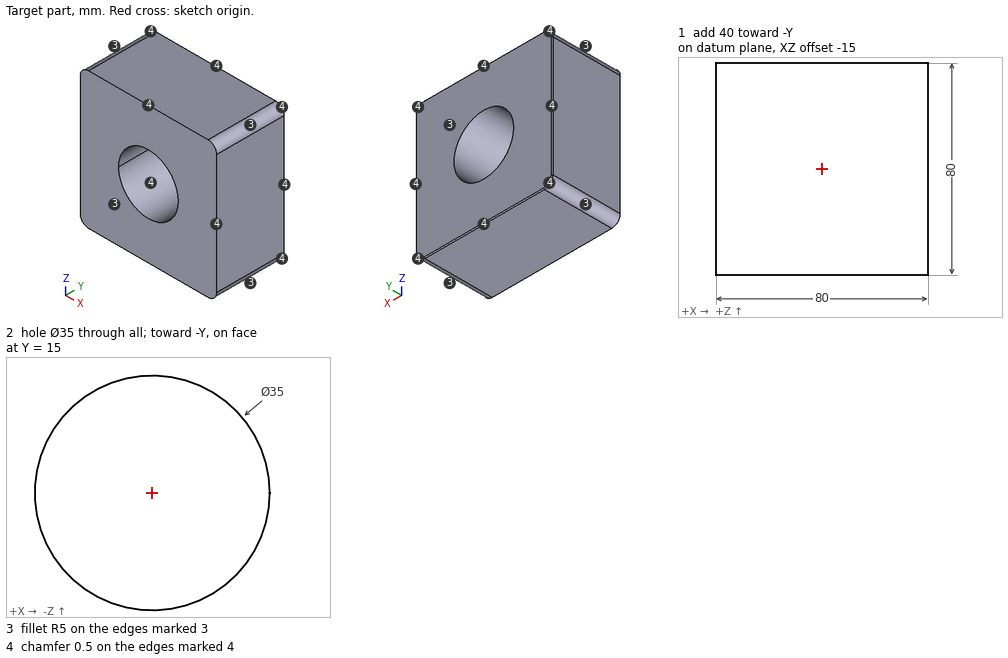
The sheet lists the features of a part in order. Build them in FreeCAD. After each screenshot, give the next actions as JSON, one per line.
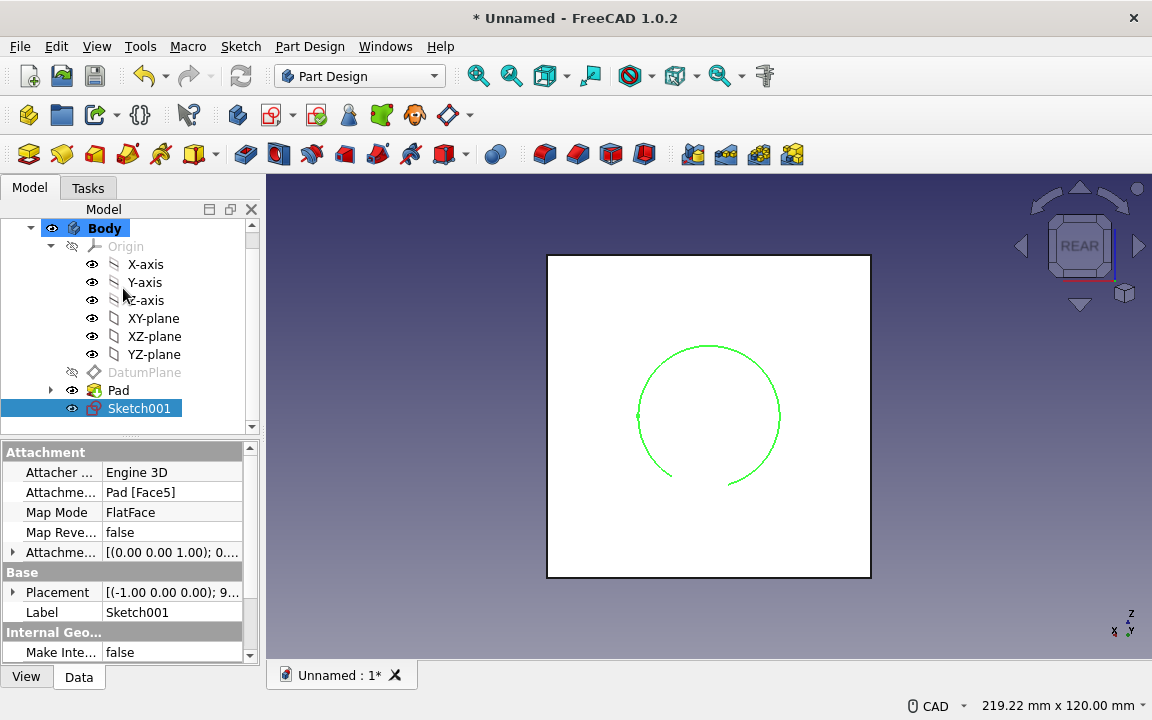
{"action": "left_click", "coordinate": [279, 154]}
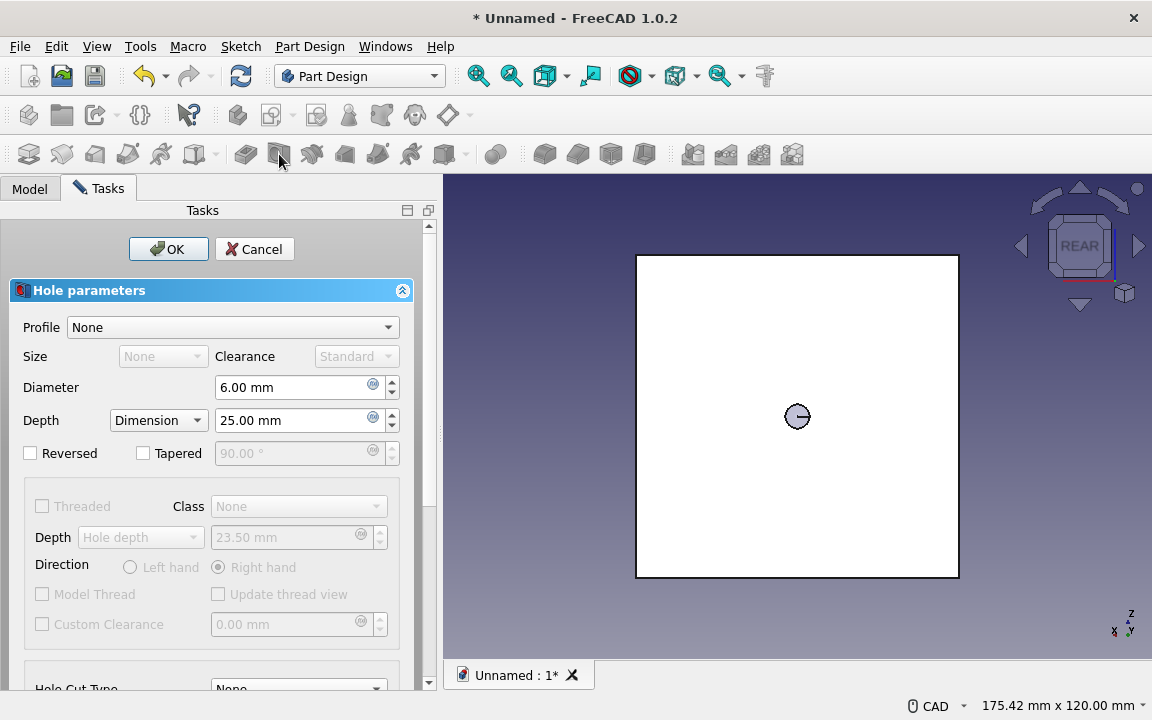
{"action": "triple_click", "coordinate": [300, 388]}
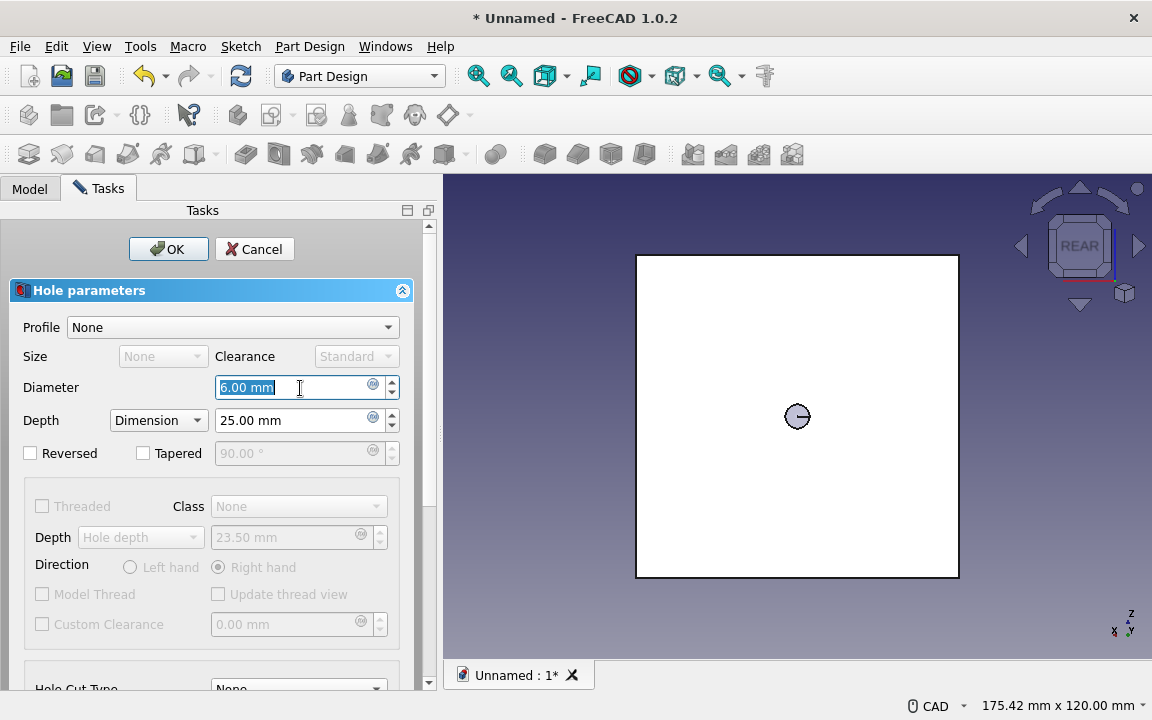
{"action": "type", "text": "35"}
{"action": "key", "text": "Tab"}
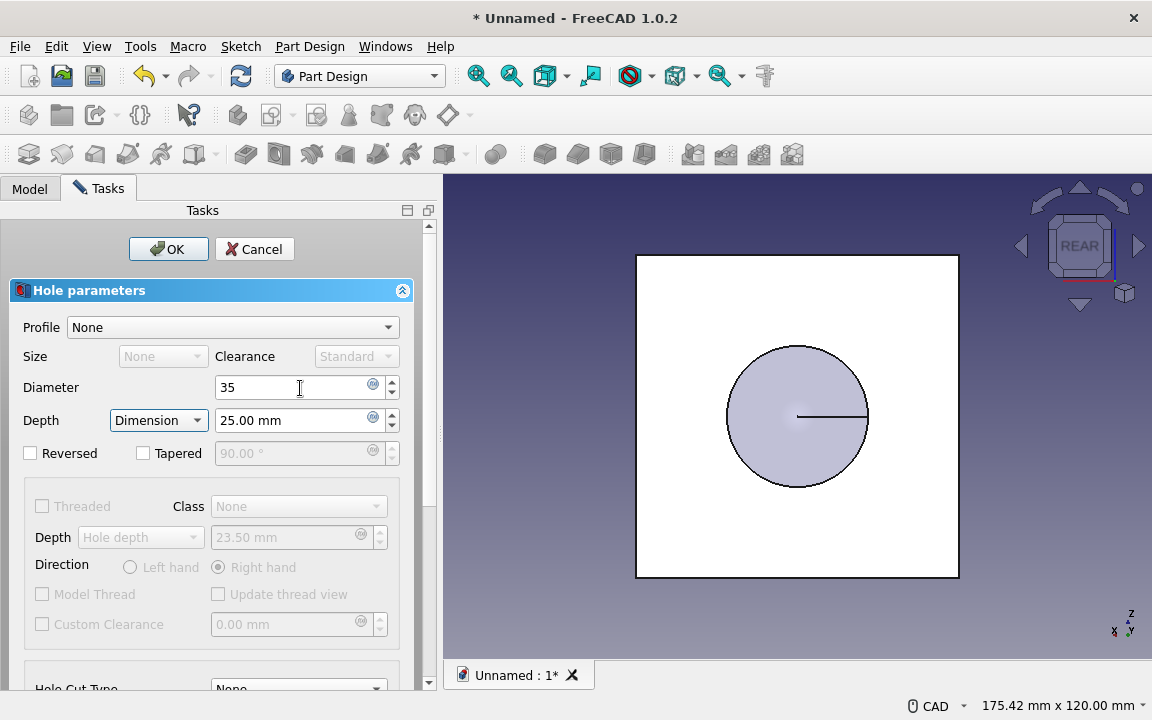
{"action": "left_click", "coordinate": [160, 420]}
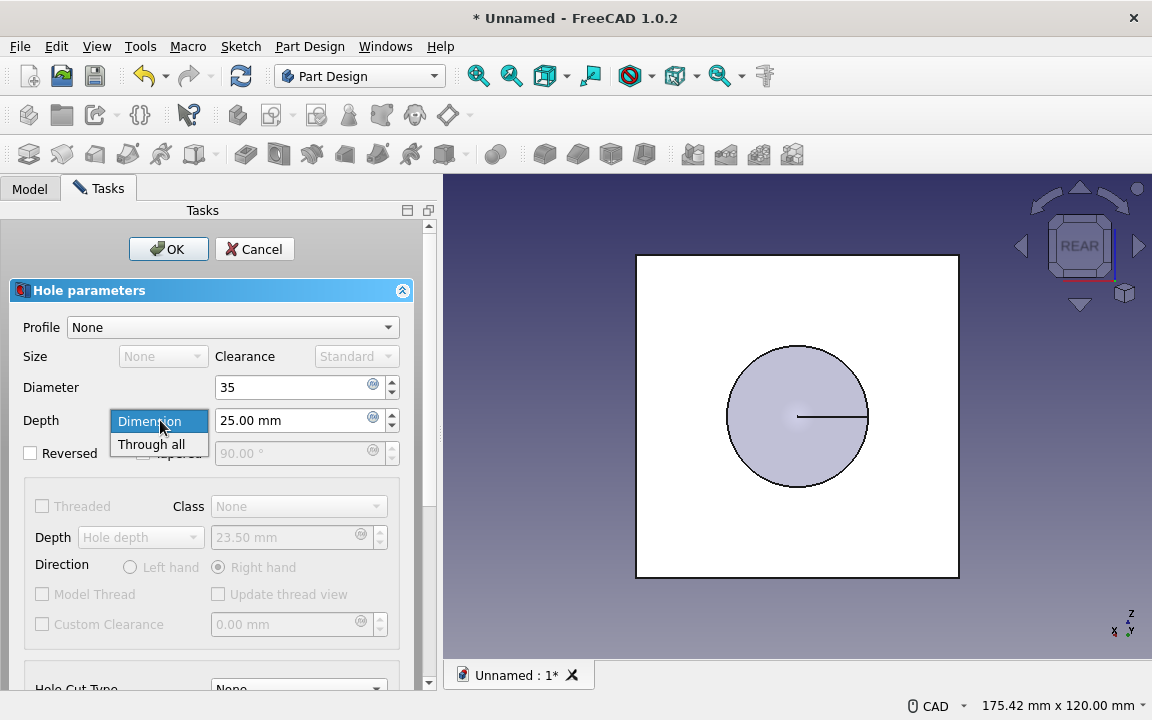
{"action": "left_click", "coordinate": [158, 444]}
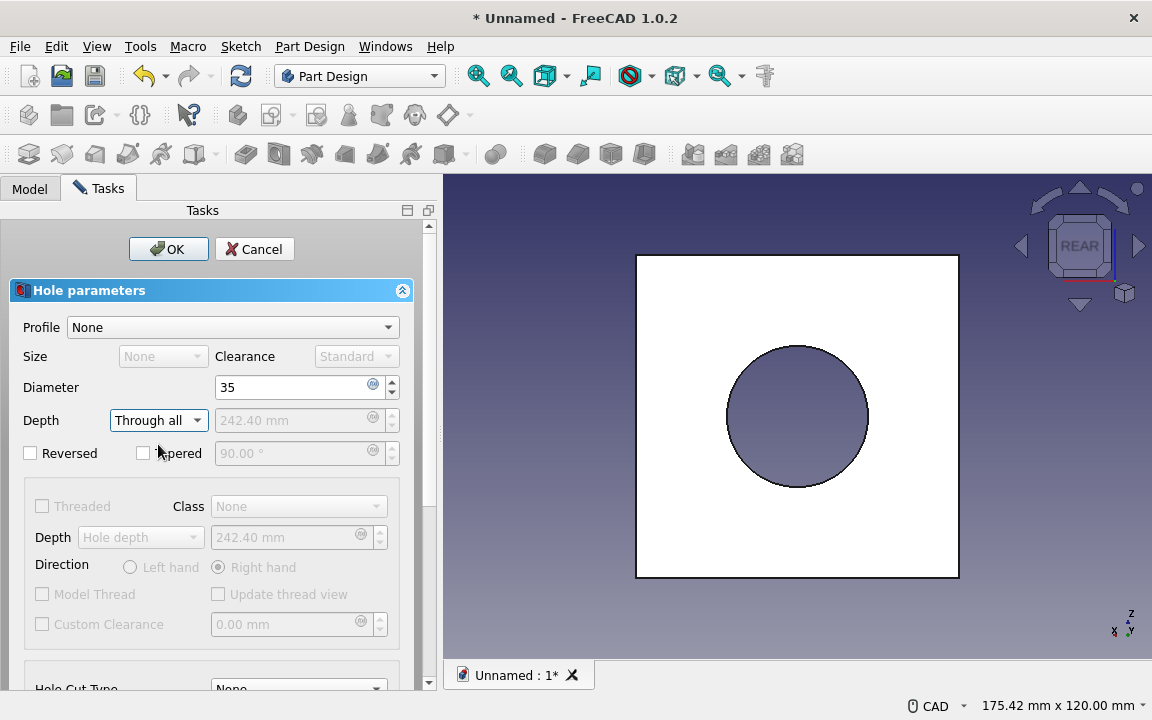
{"action": "left_click", "coordinate": [169, 249]}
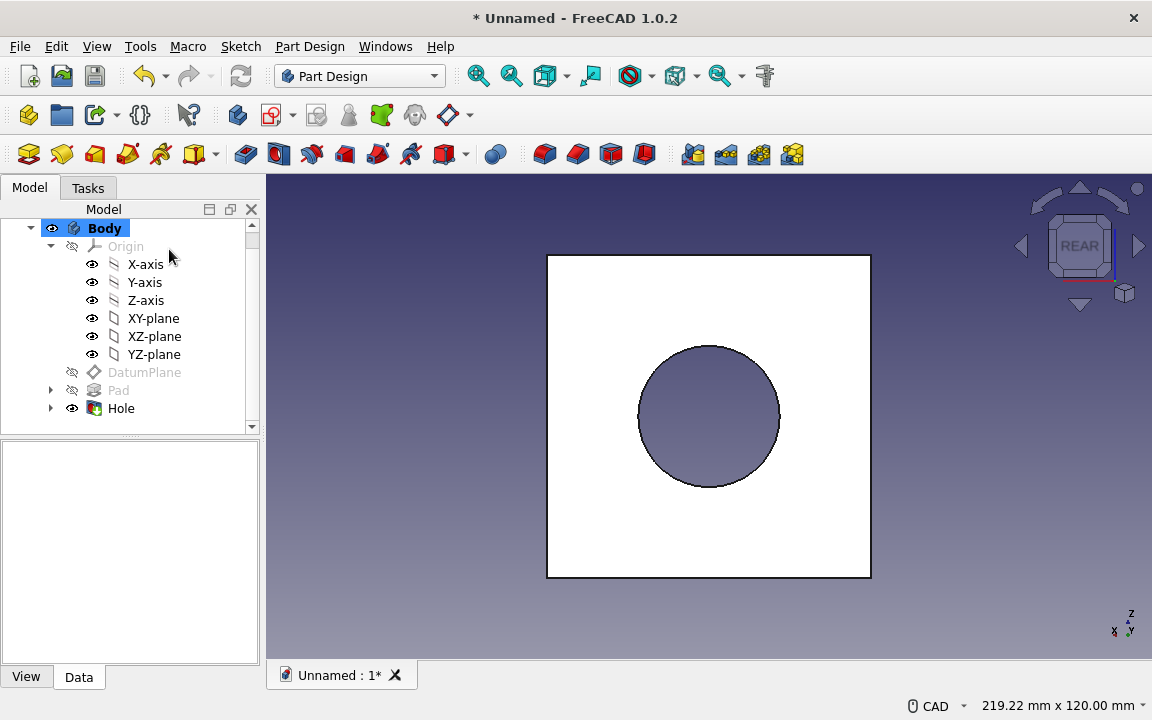
{"action": "key", "text": "0"}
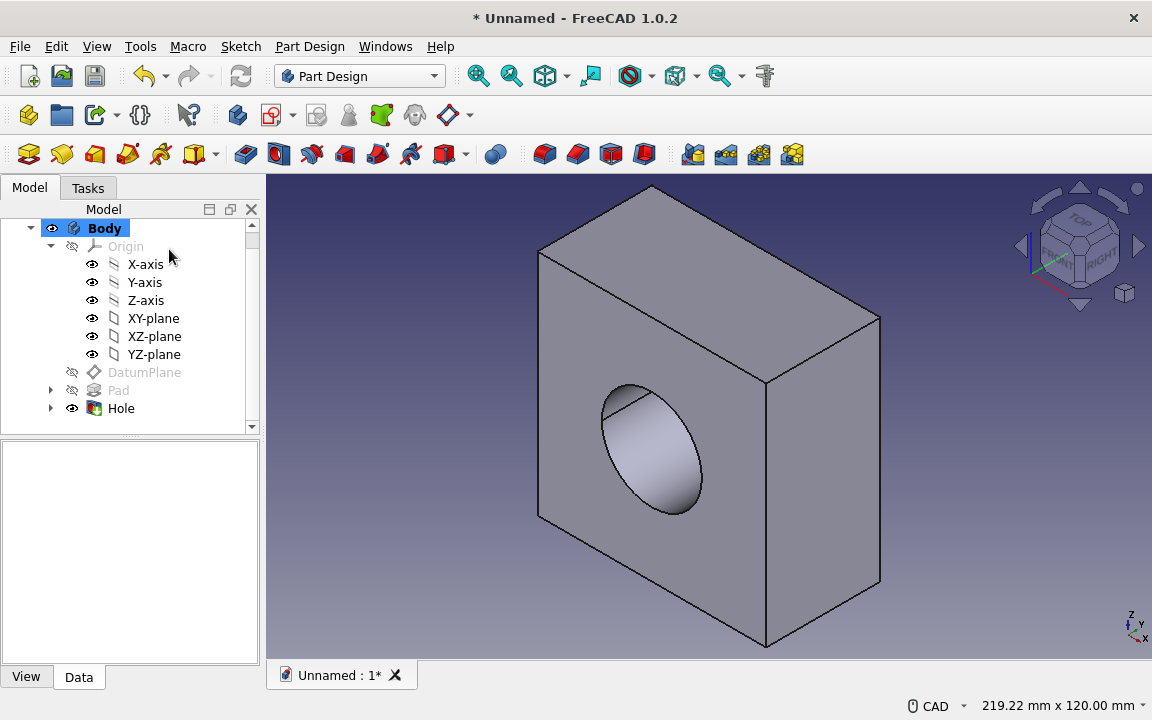
{"action": "left_click", "coordinate": [823, 349]}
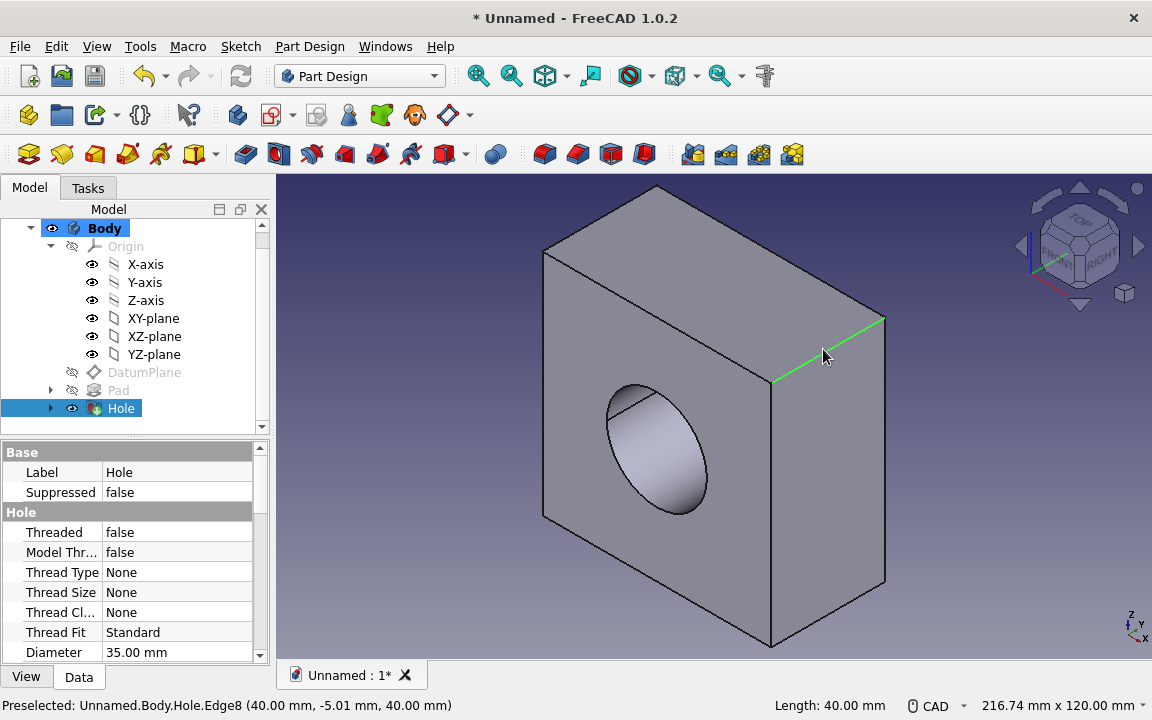
{"action": "key", "text": "2"}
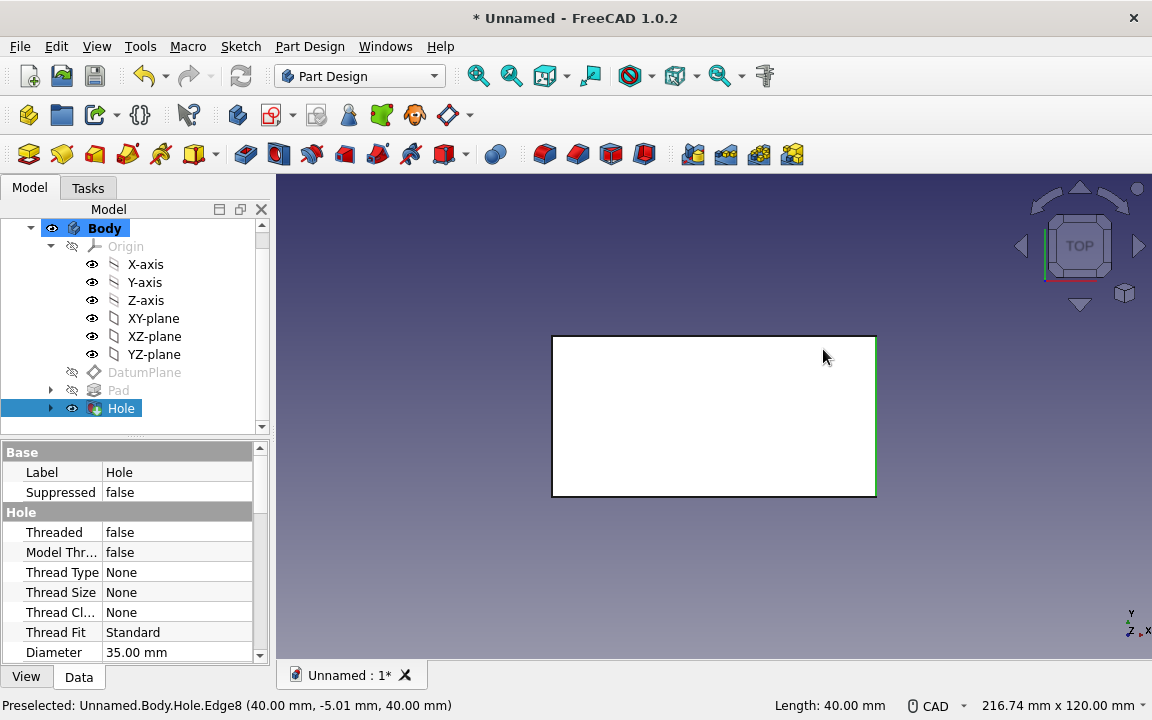
{"action": "left_click", "coordinate": [479, 76]}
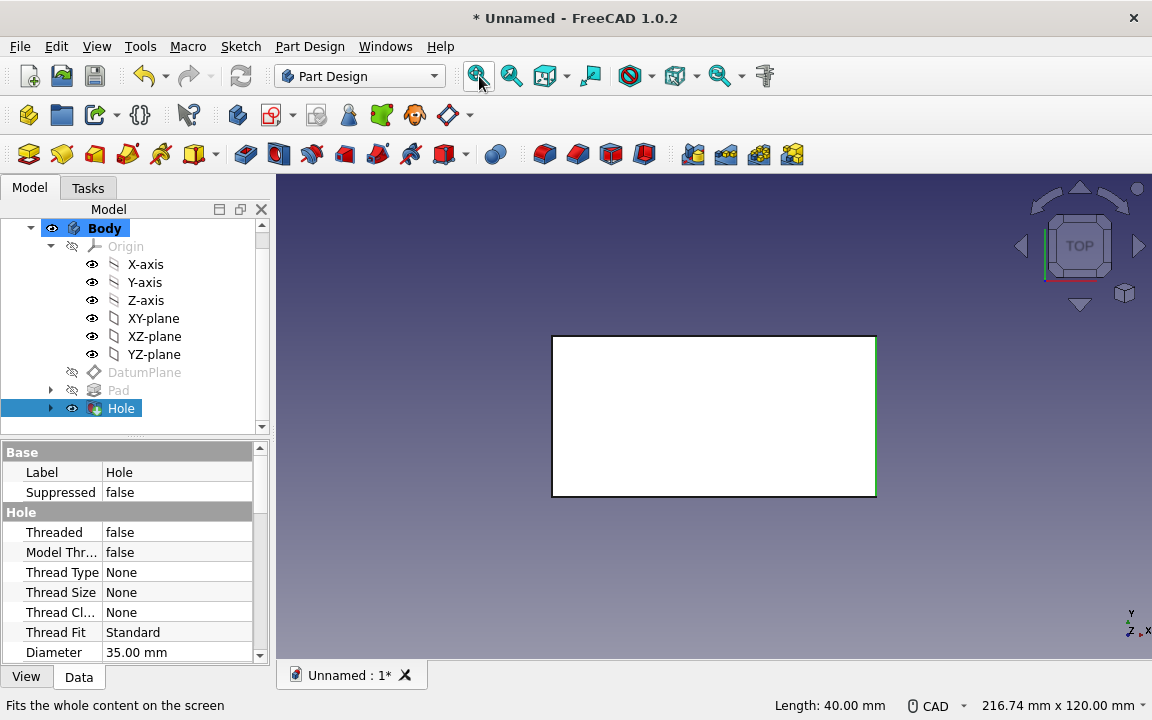
{"action": "left_click", "coordinate": [552, 415], "text": "ctrl"}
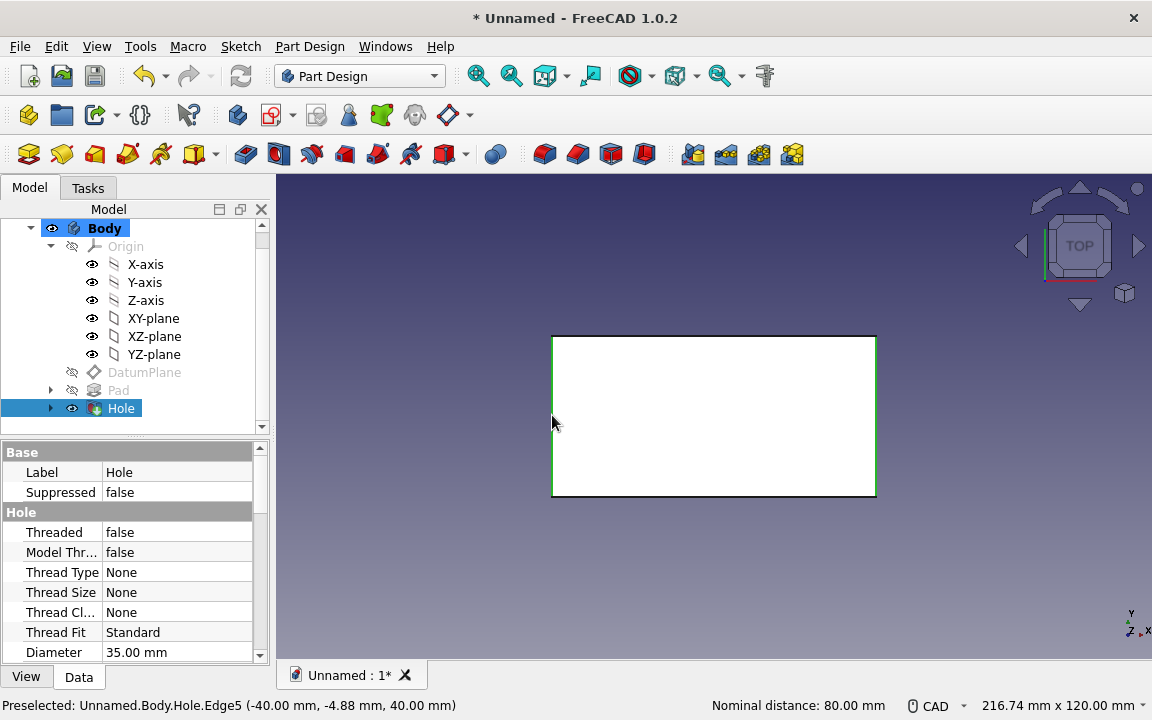
{"action": "key", "text": "1"}